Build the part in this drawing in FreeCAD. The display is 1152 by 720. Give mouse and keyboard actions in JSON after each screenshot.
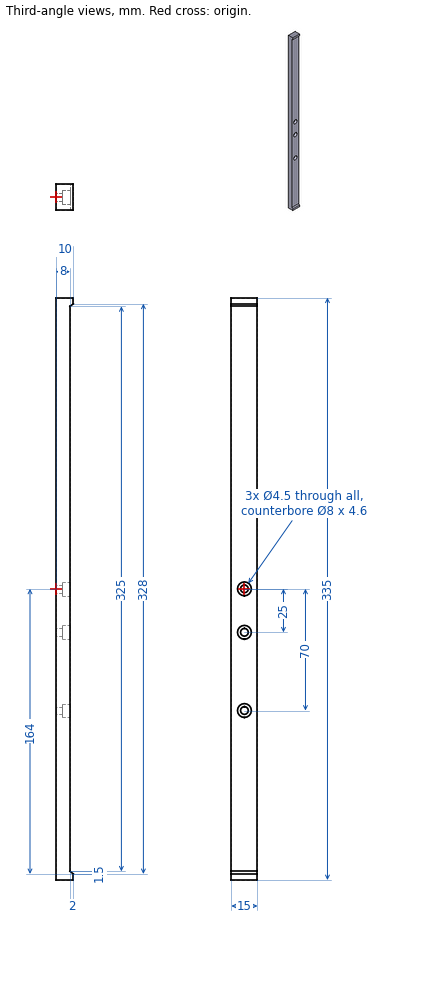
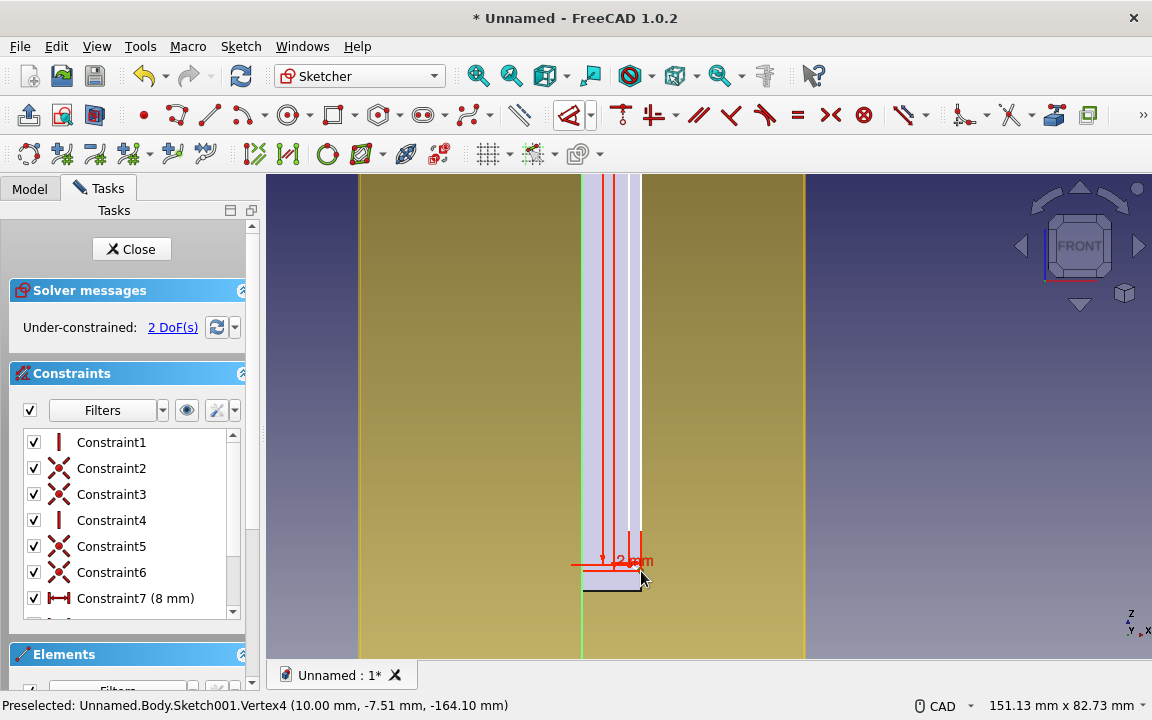
{"action": "left_click", "coordinate": [590, 116]}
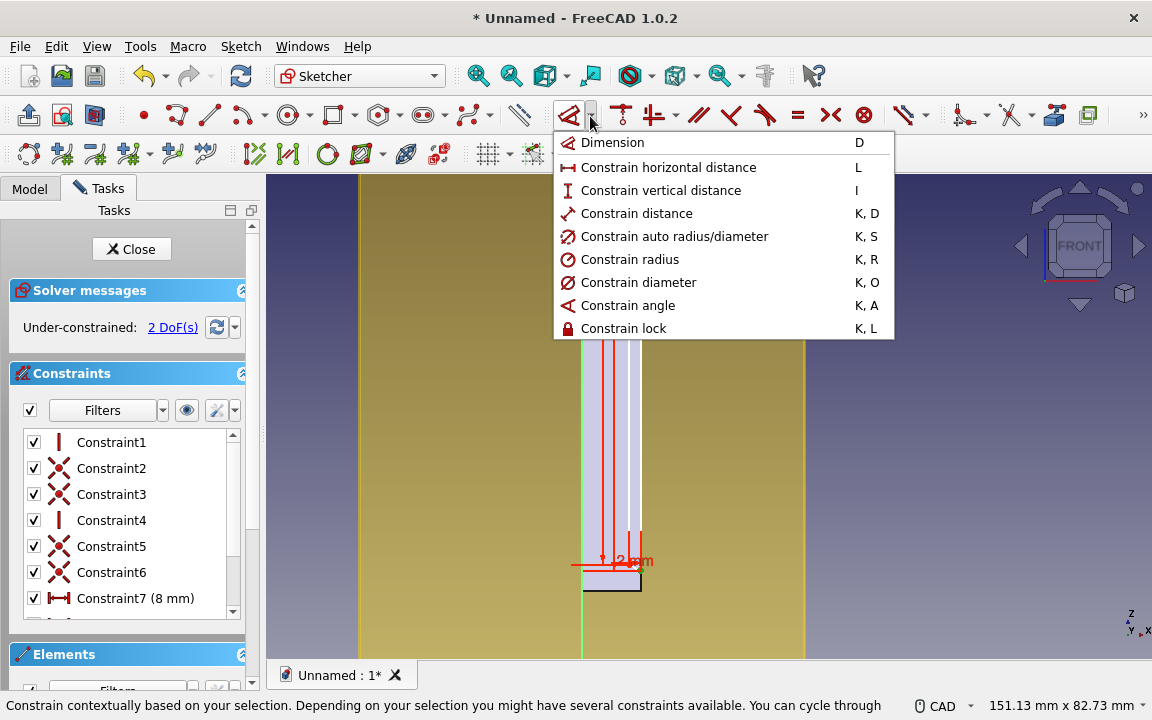
{"action": "left_click", "coordinate": [724, 190]}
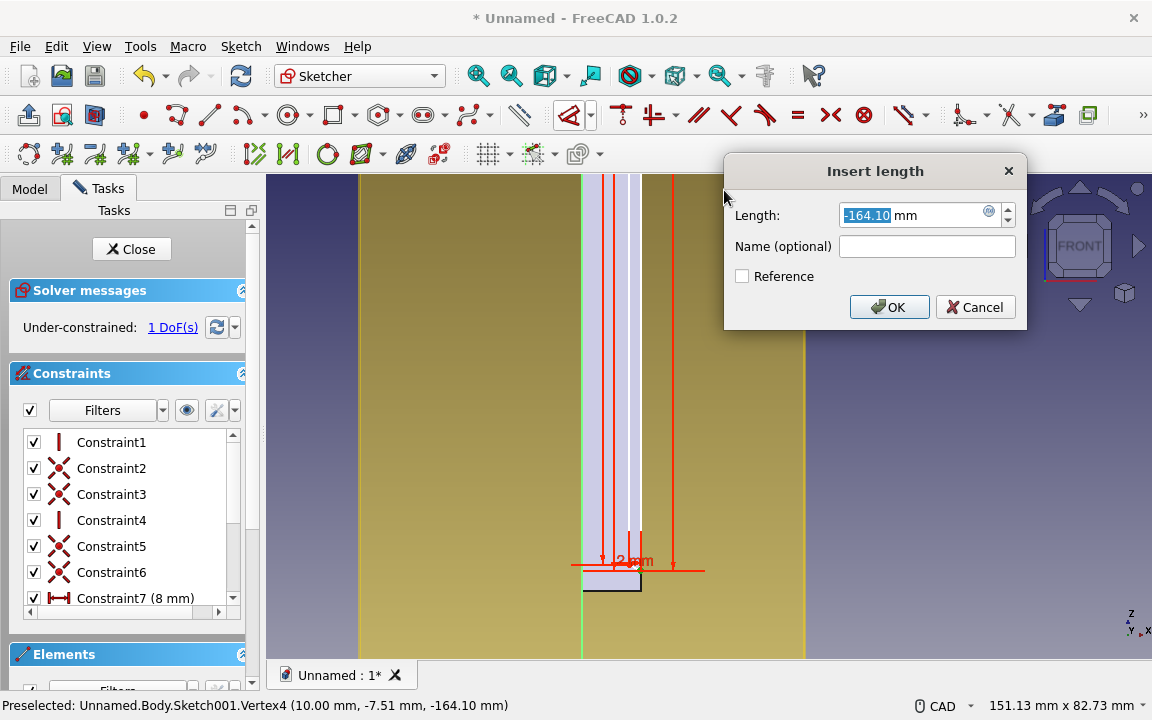
{"action": "type", "text": "-164"}
{"action": "key", "text": "Return"}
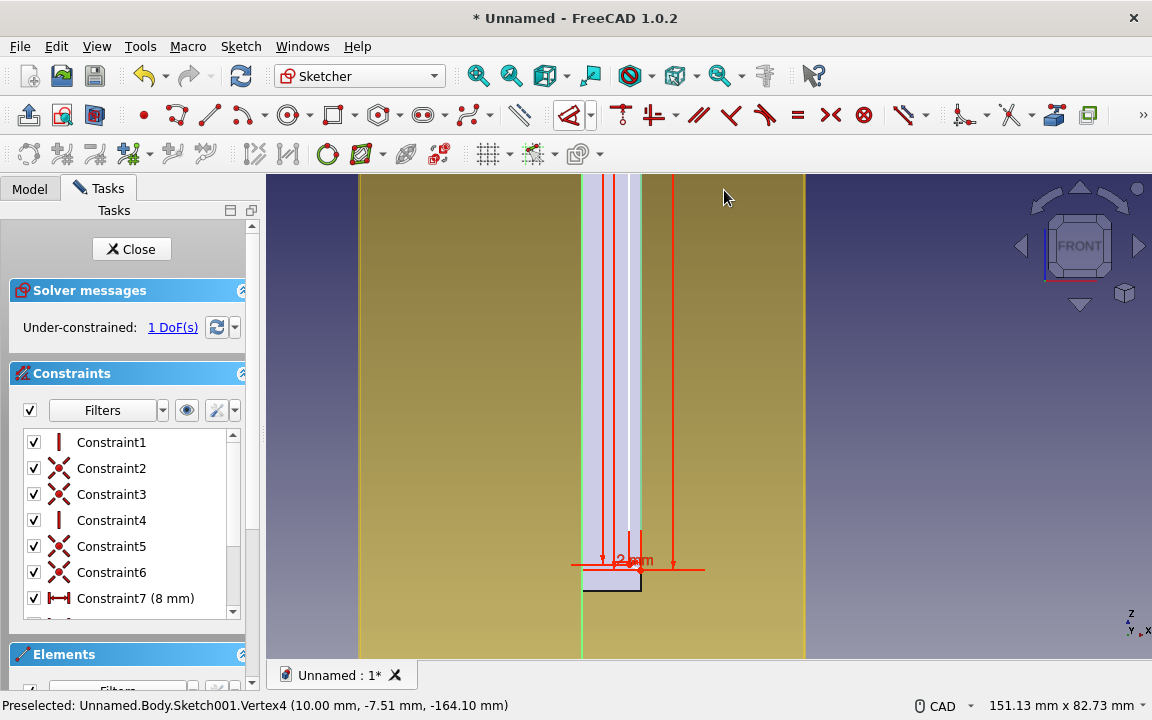
{"action": "scroll", "coordinate": [635, 568], "scroll_direction": "up", "scroll_amount": 8}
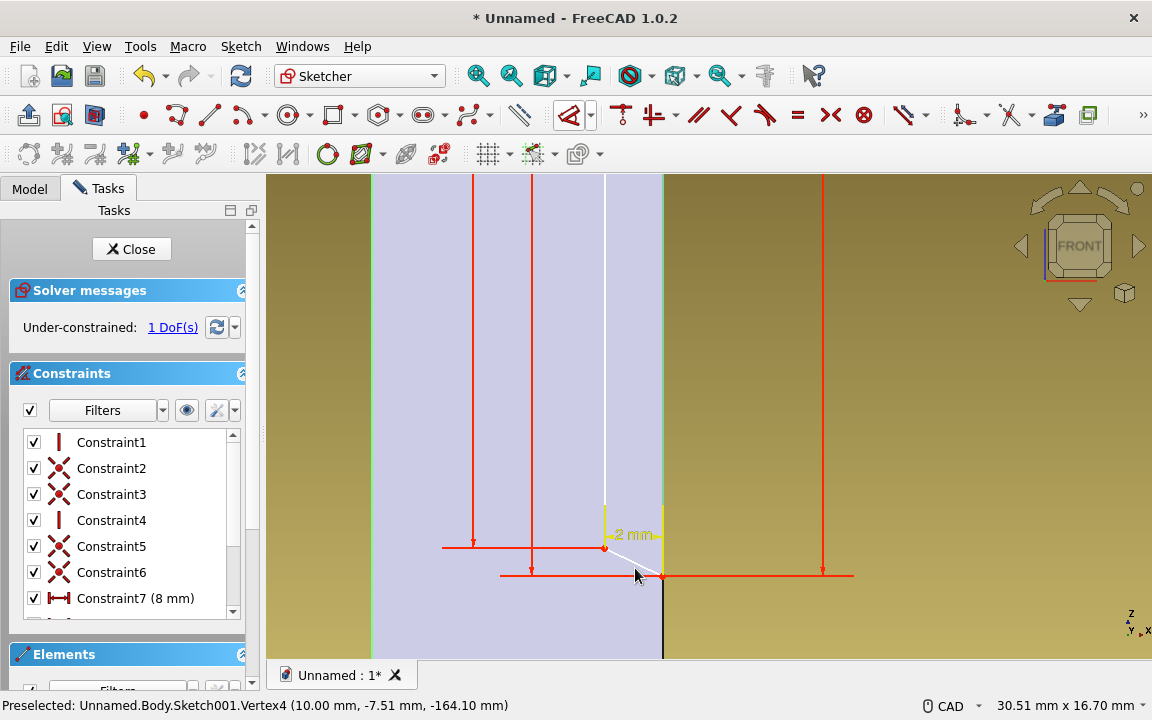
{"action": "left_click", "coordinate": [634, 562]}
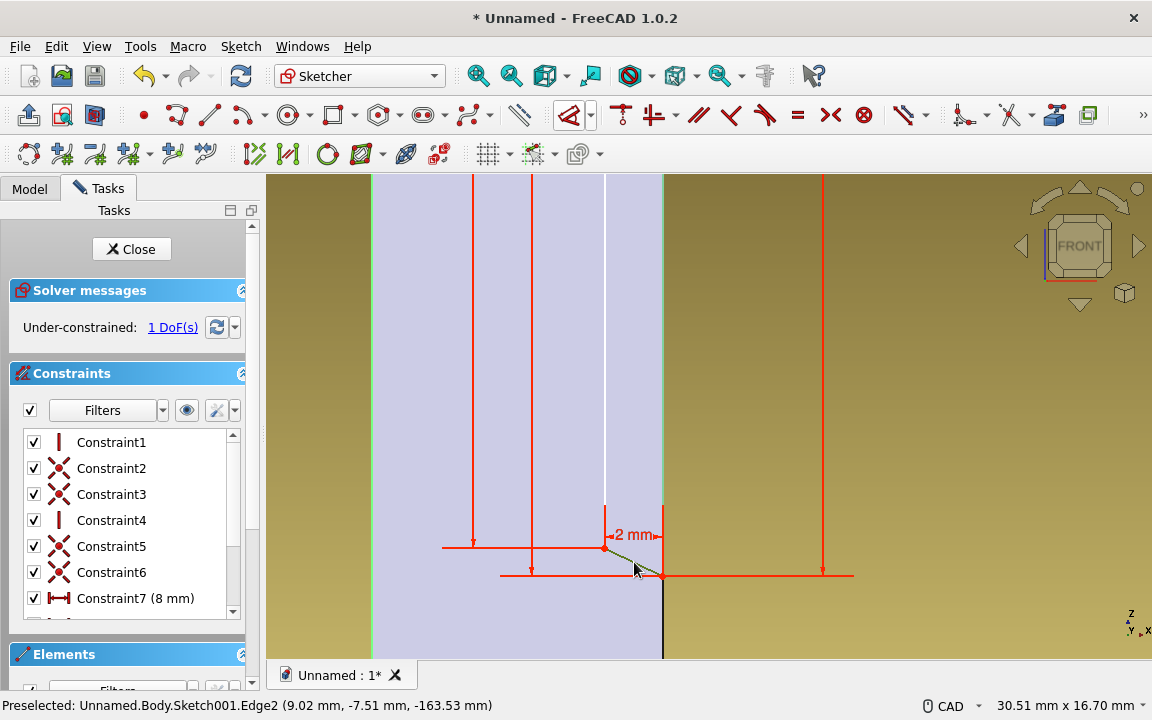
{"action": "left_click", "coordinate": [590, 116]}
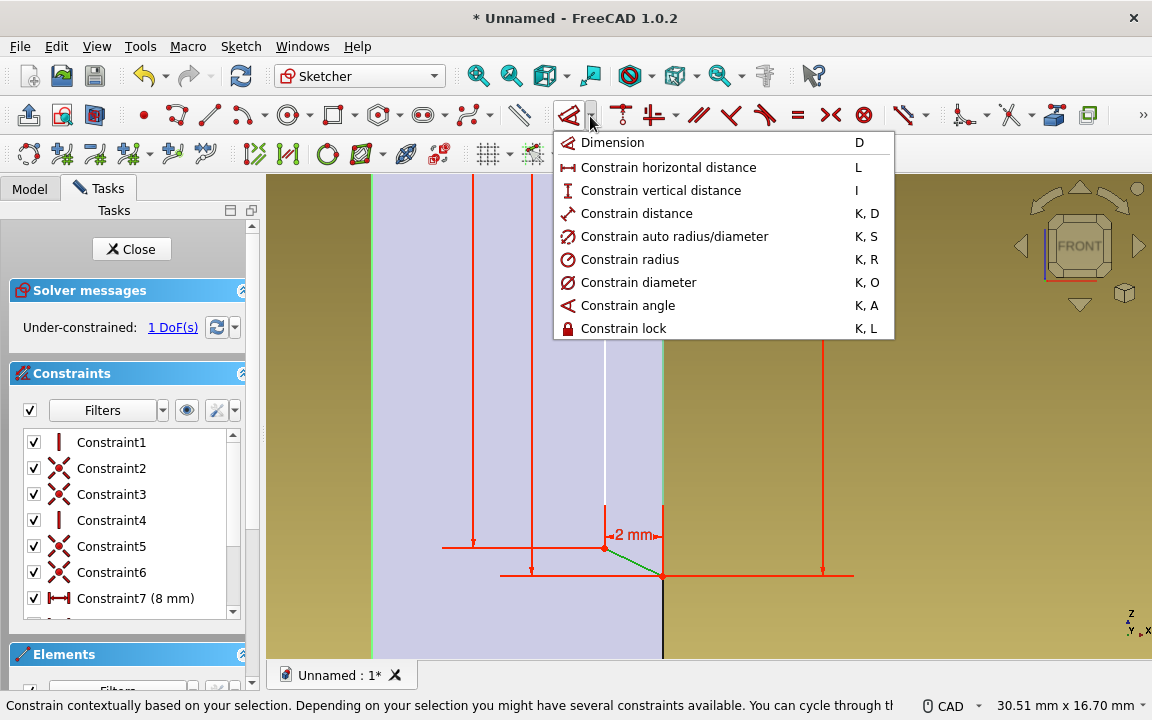
{"action": "left_click", "coordinate": [724, 190]}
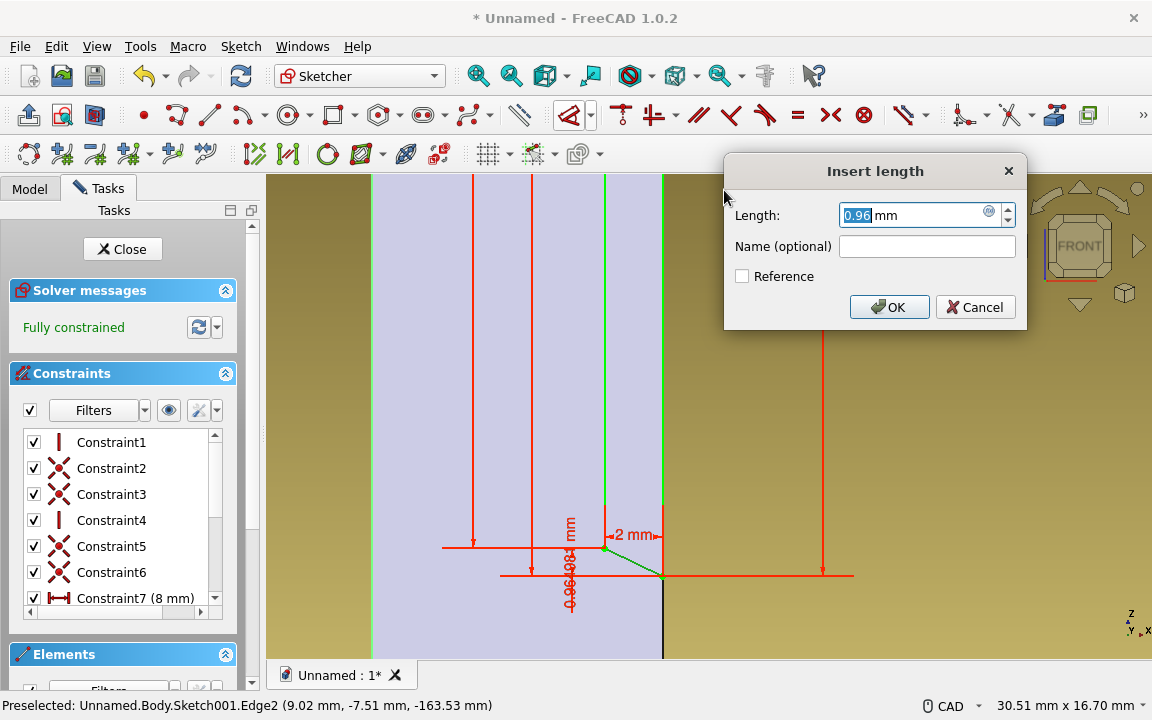
{"action": "type", "text": "1.5"}
{"action": "key", "text": "Return"}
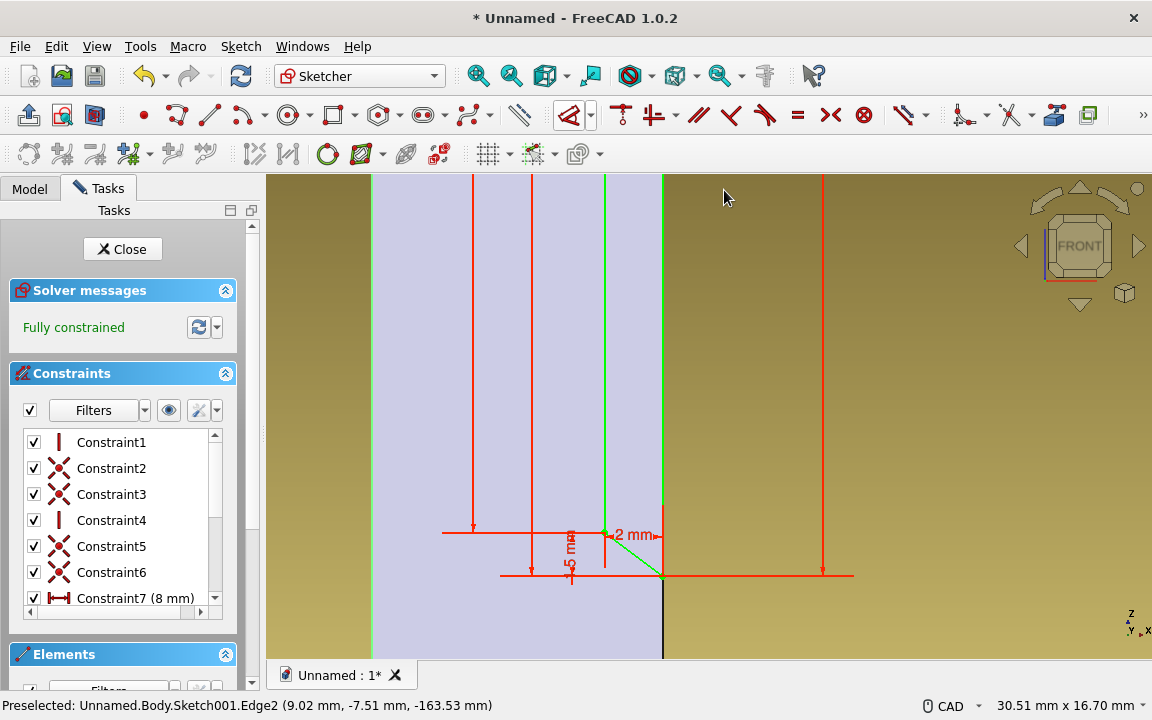
{"action": "left_click", "coordinate": [123, 249]}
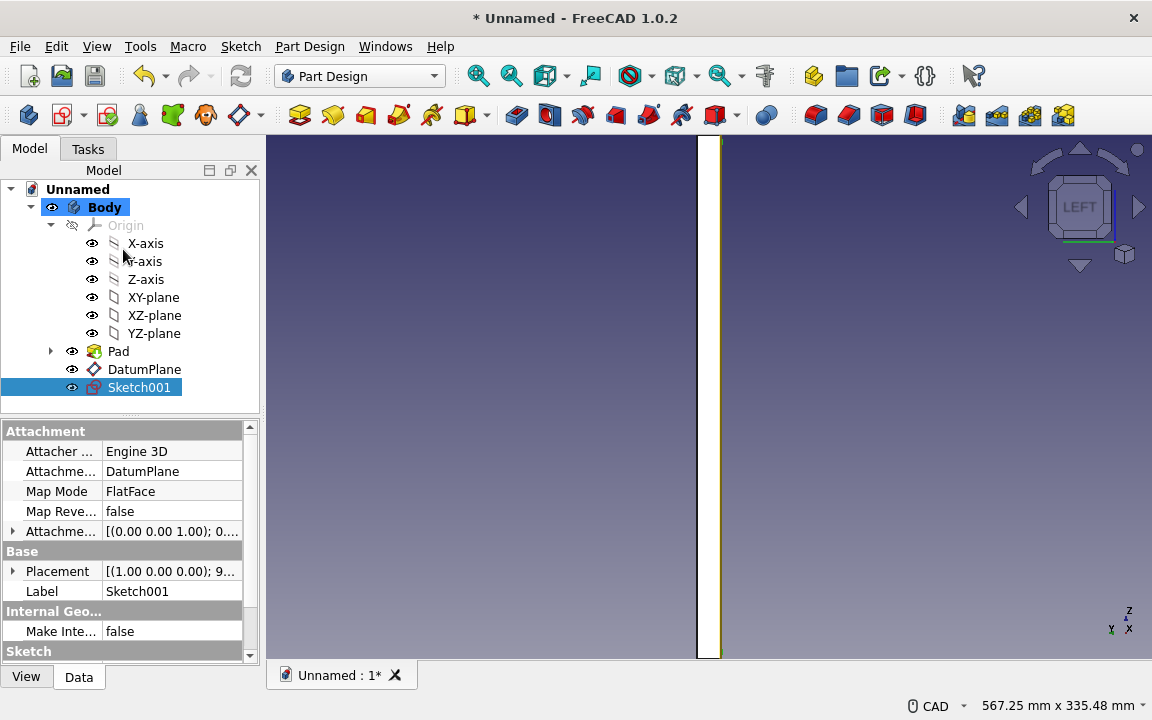
{"action": "left_click", "coordinate": [517, 116]}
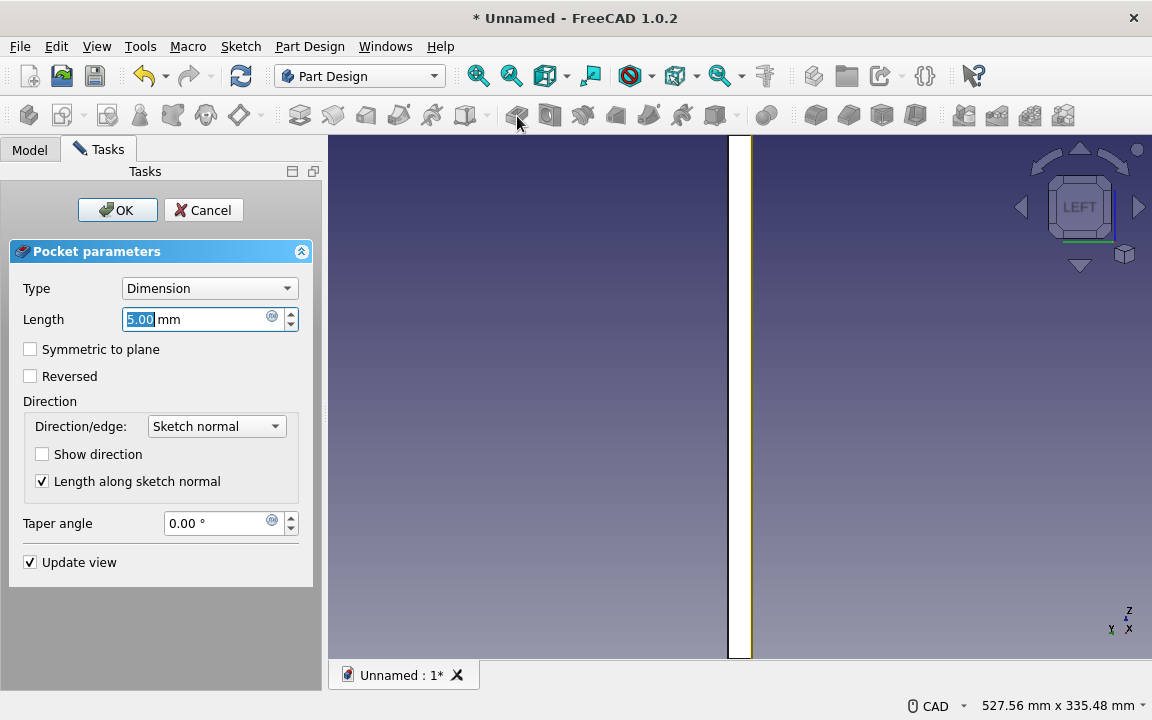
{"action": "left_click", "coordinate": [210, 288]}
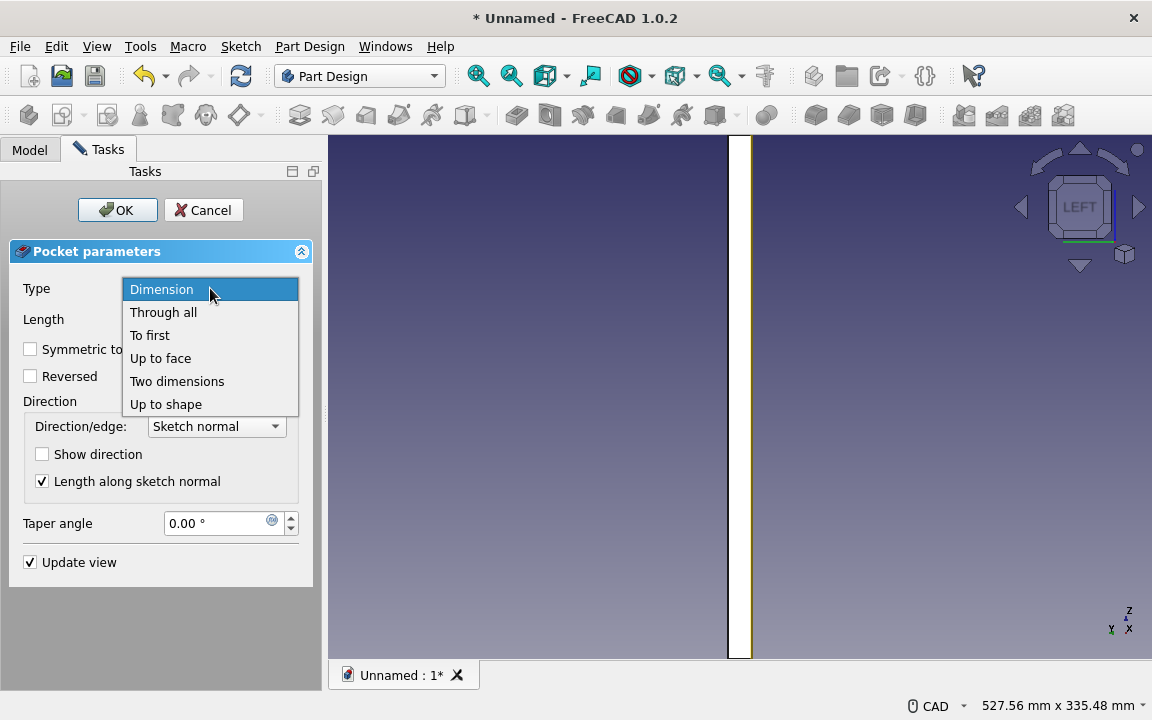
{"action": "left_click", "coordinate": [208, 312]}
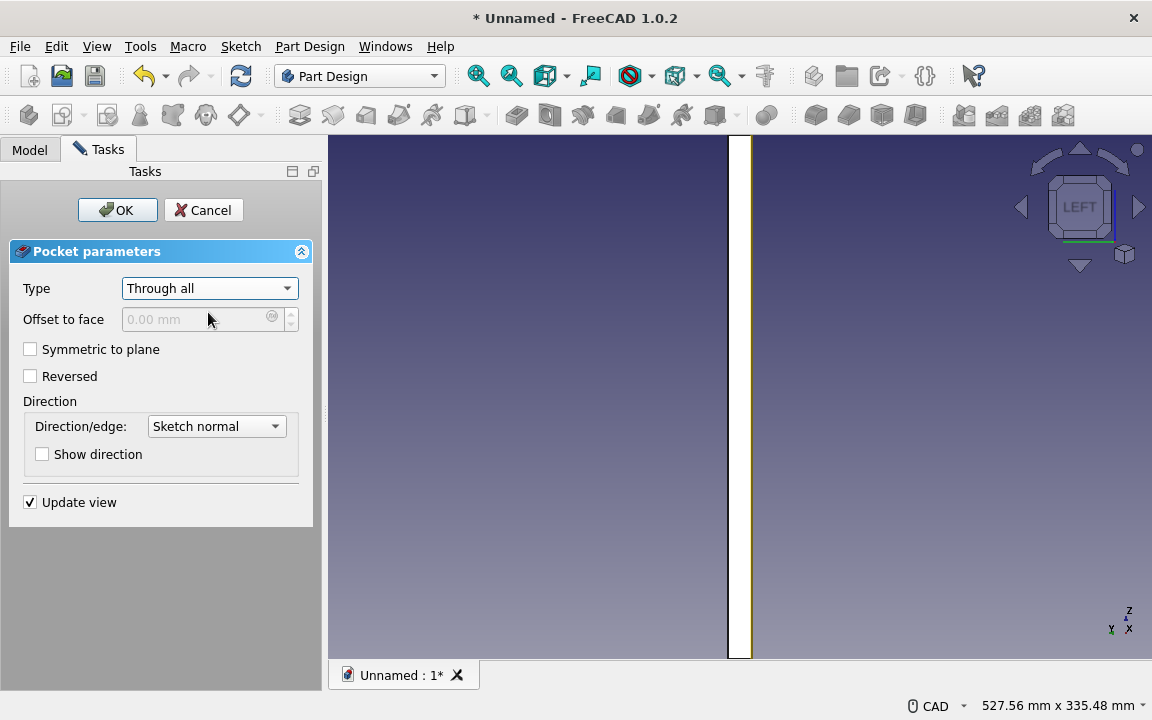
{"action": "left_click", "coordinate": [118, 210]}